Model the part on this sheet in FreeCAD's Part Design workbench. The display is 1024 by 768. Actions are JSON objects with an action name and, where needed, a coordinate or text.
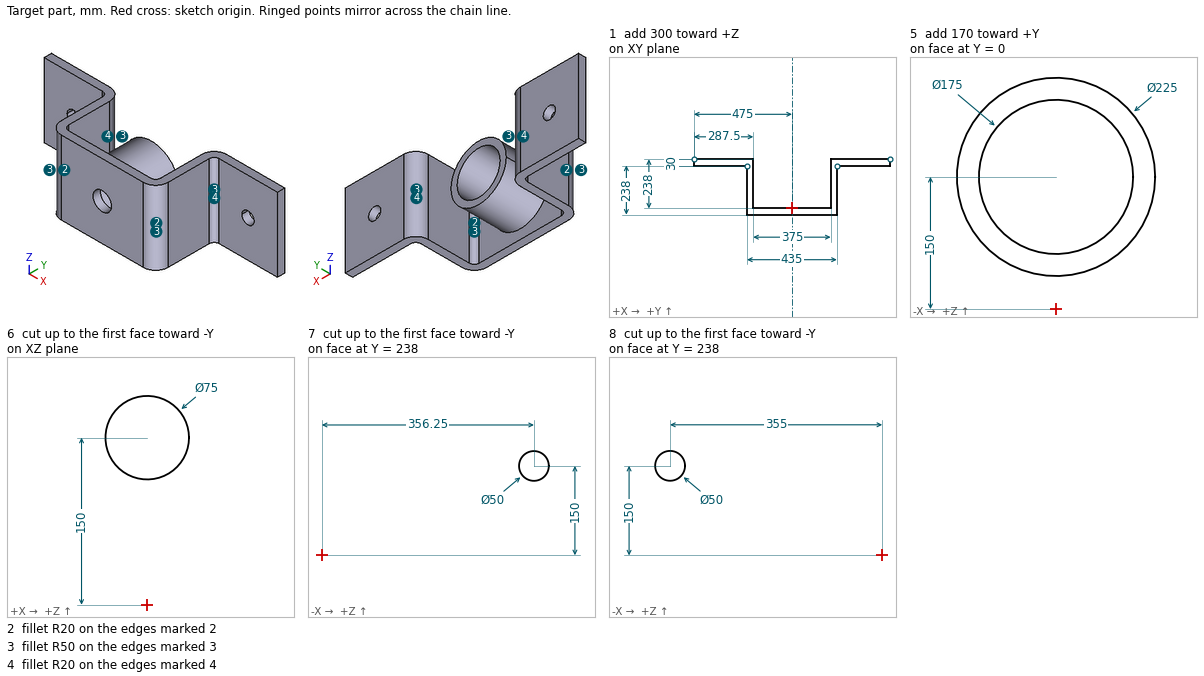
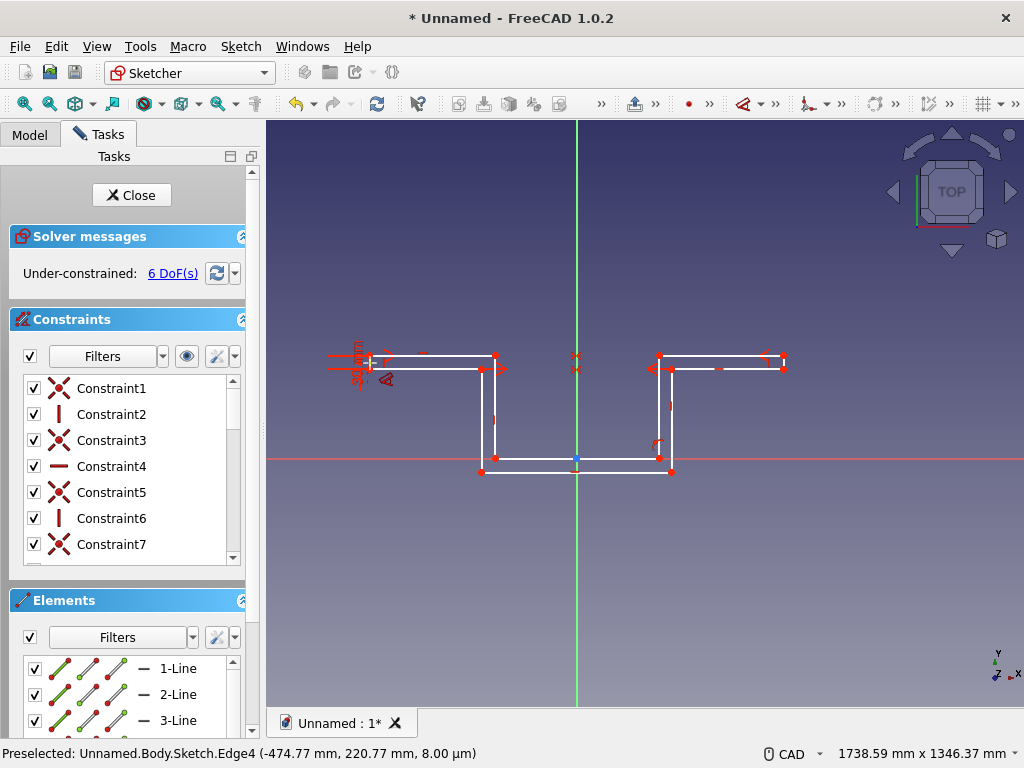
{"action": "left_click", "coordinate": [610, 459]}
{"action": "left_click", "coordinate": [539, 493]}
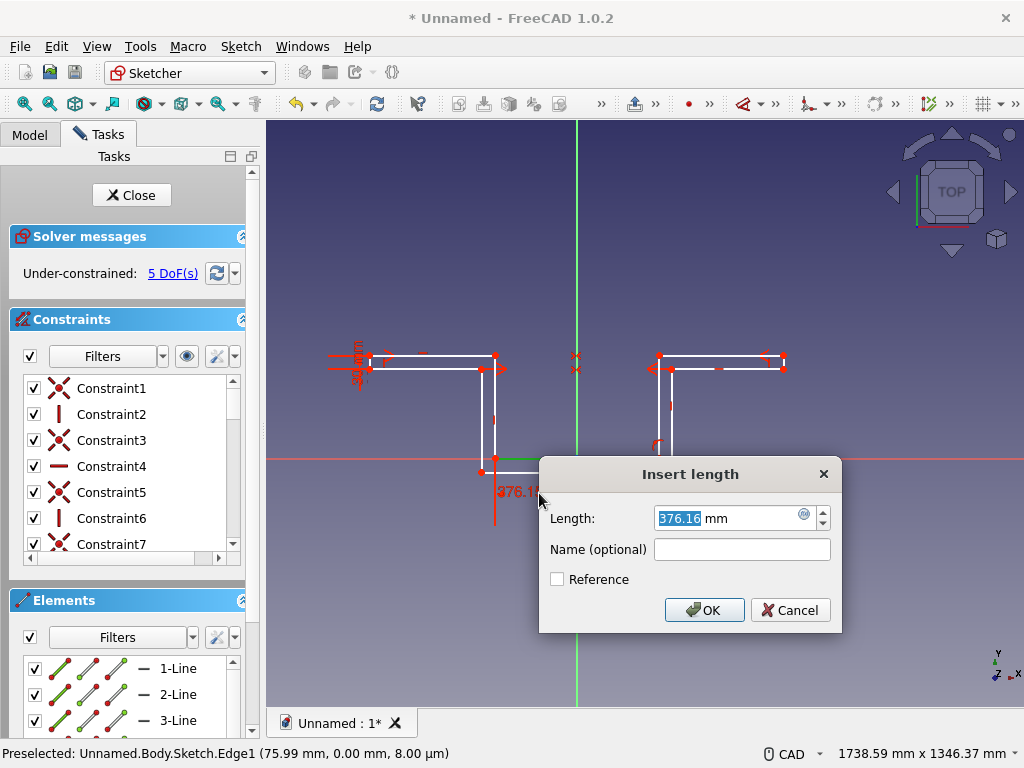
{"action": "type", "text": "375"}
{"action": "key", "text": "Return"}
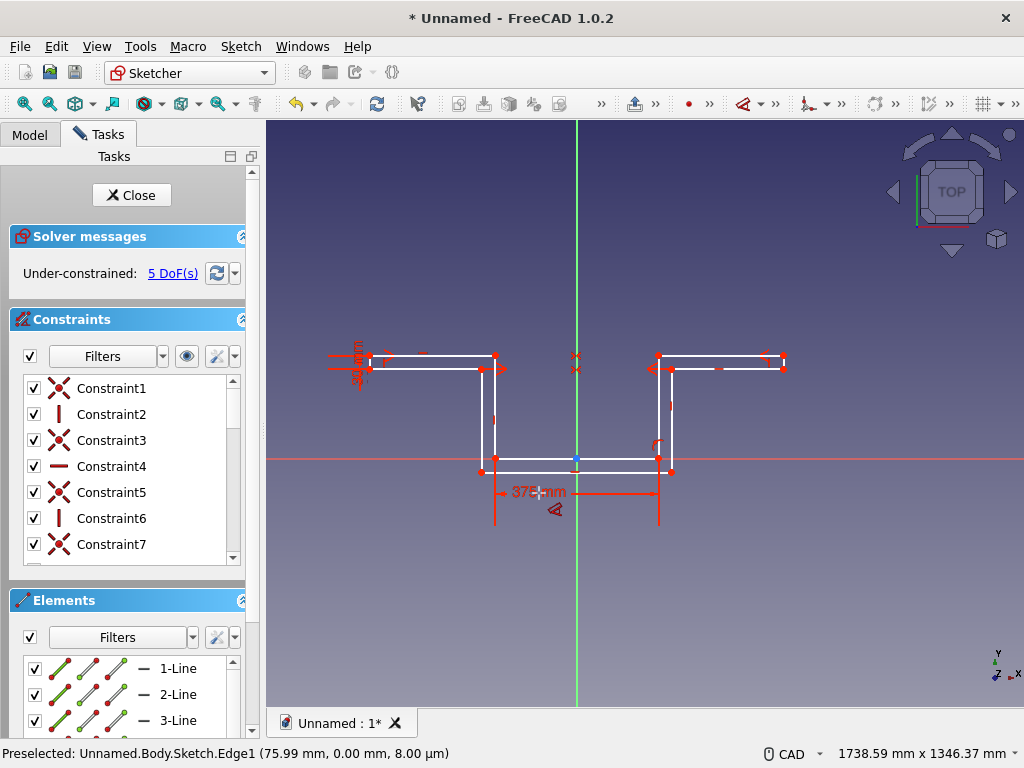
{"action": "left_click", "coordinate": [495, 428]}
{"action": "left_click", "coordinate": [461, 407]}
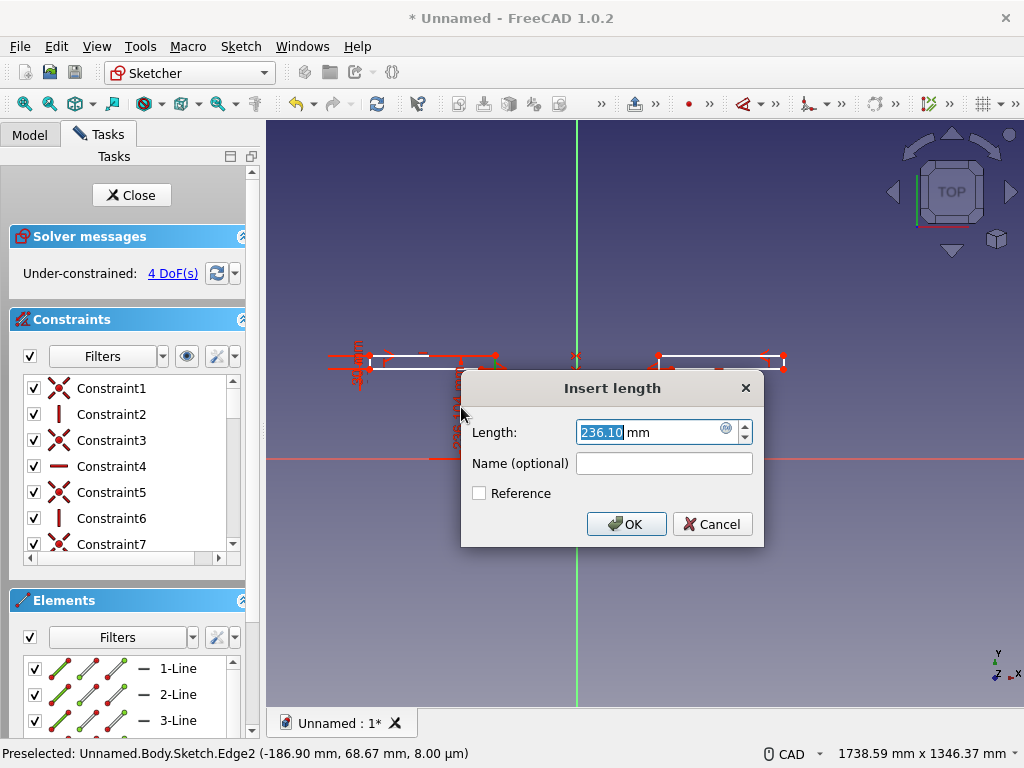
{"action": "type", "text": "238"}
{"action": "key", "text": "Return"}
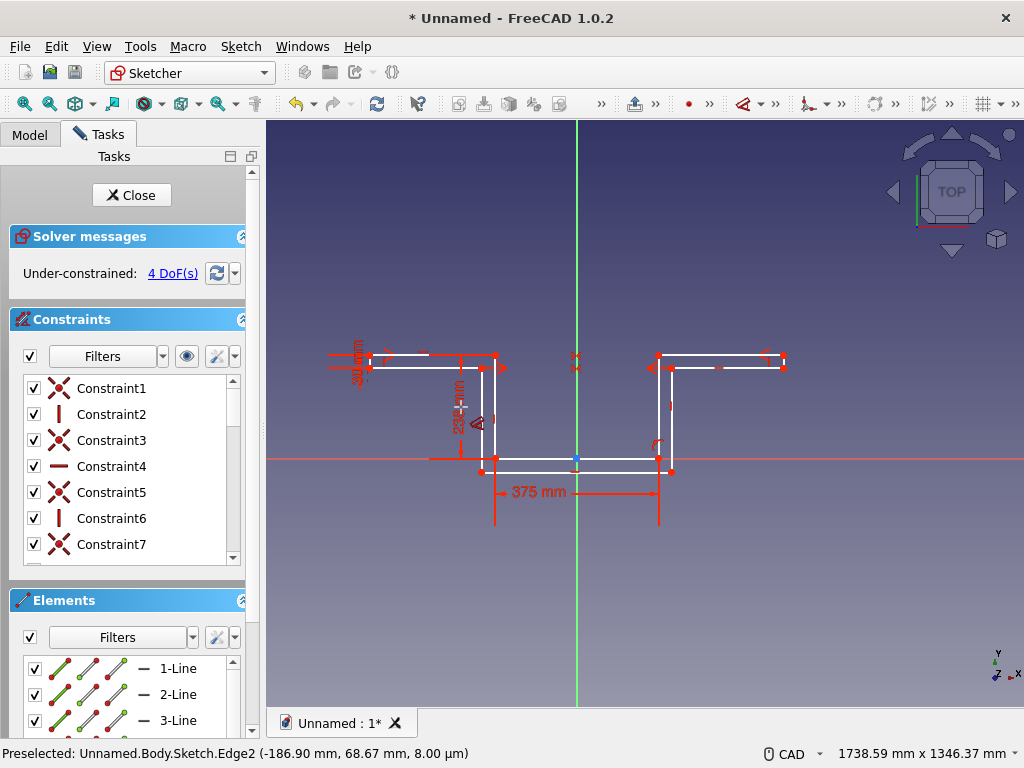
{"action": "left_click", "coordinate": [482, 400]}
{"action": "left_click", "coordinate": [448, 445]}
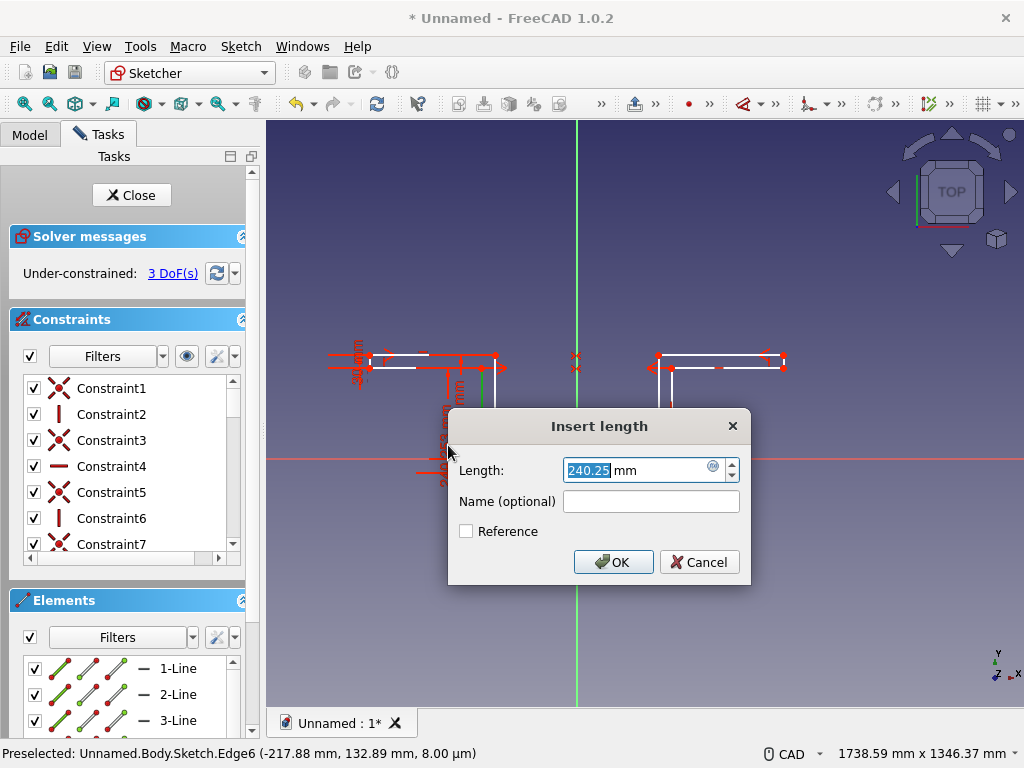
{"action": "type", "text": "238"}
{"action": "key", "text": "Return"}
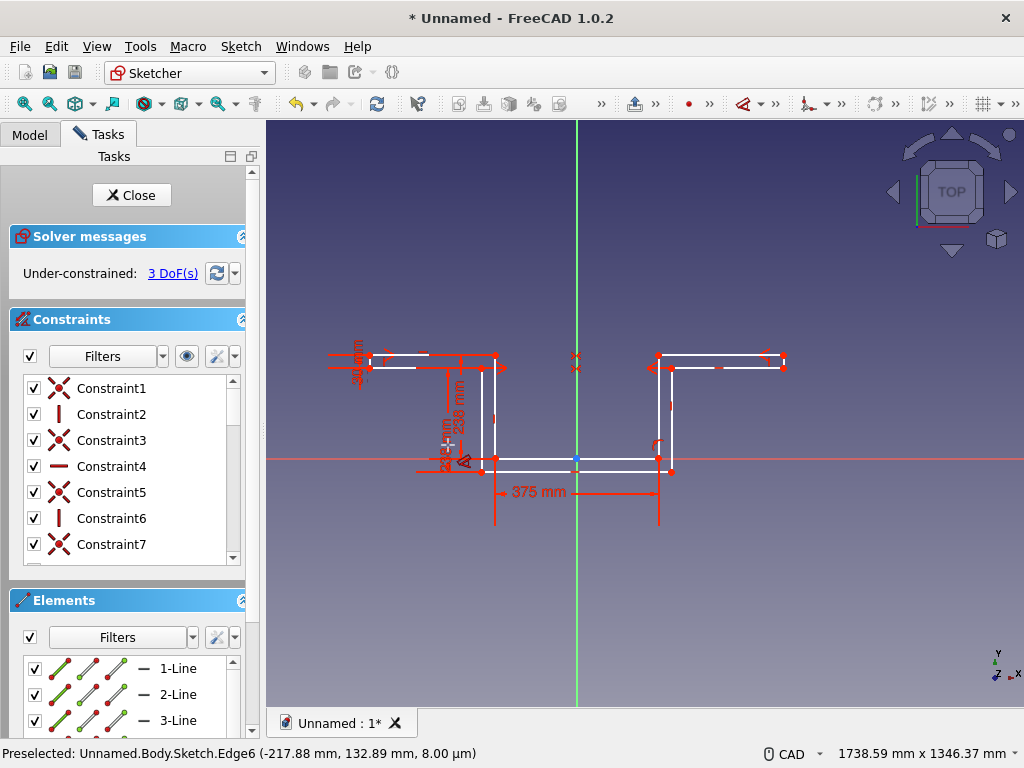
{"action": "left_click", "coordinate": [539, 472]}
{"action": "left_click", "coordinate": [621, 506]}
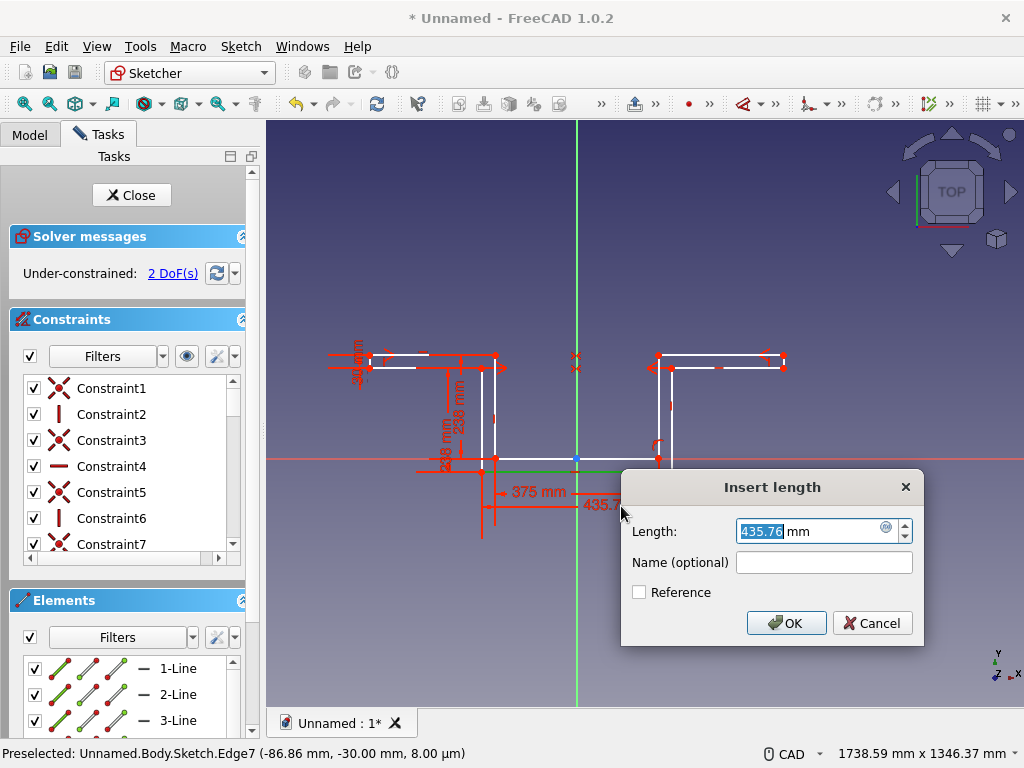
{"action": "type", "text": "435"}
{"action": "key", "text": "Return"}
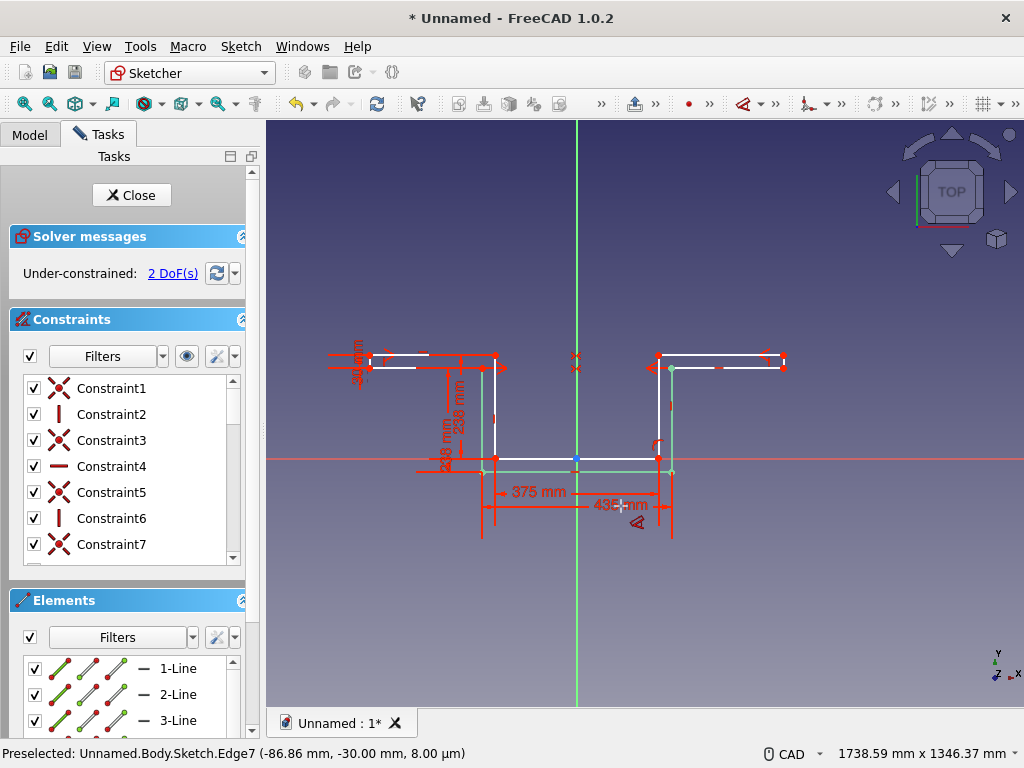
{"action": "left_click", "coordinate": [370, 355]}
{"action": "left_click", "coordinate": [473, 321]}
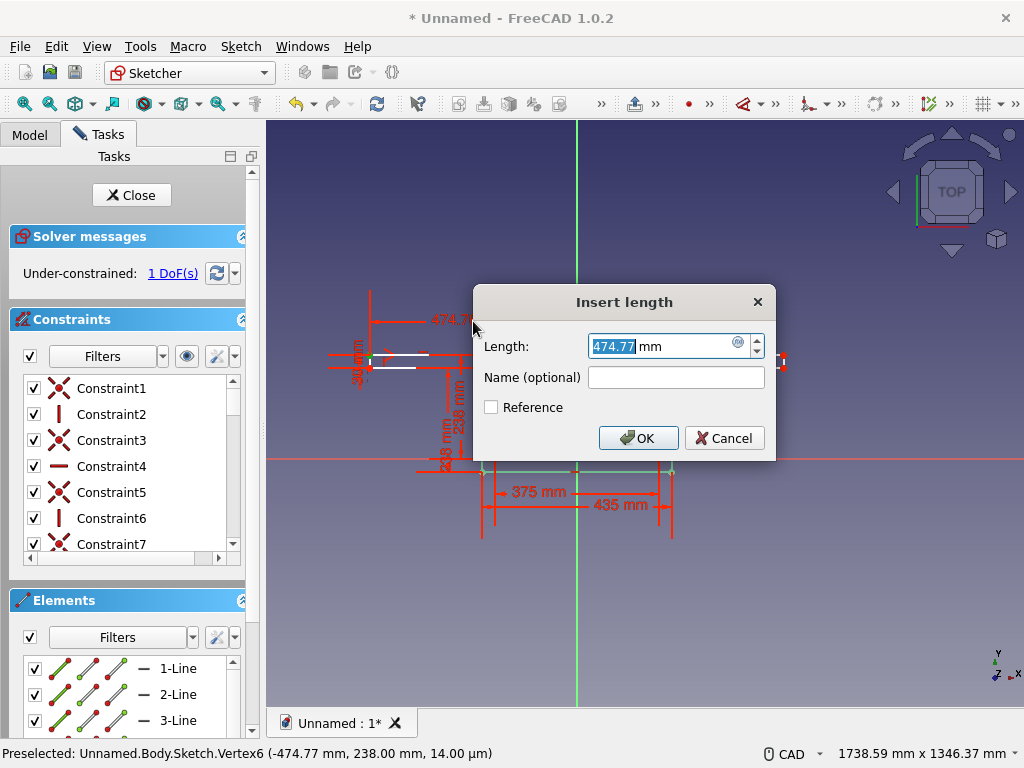
{"action": "type", "text": "475"}
{"action": "key", "text": "Return"}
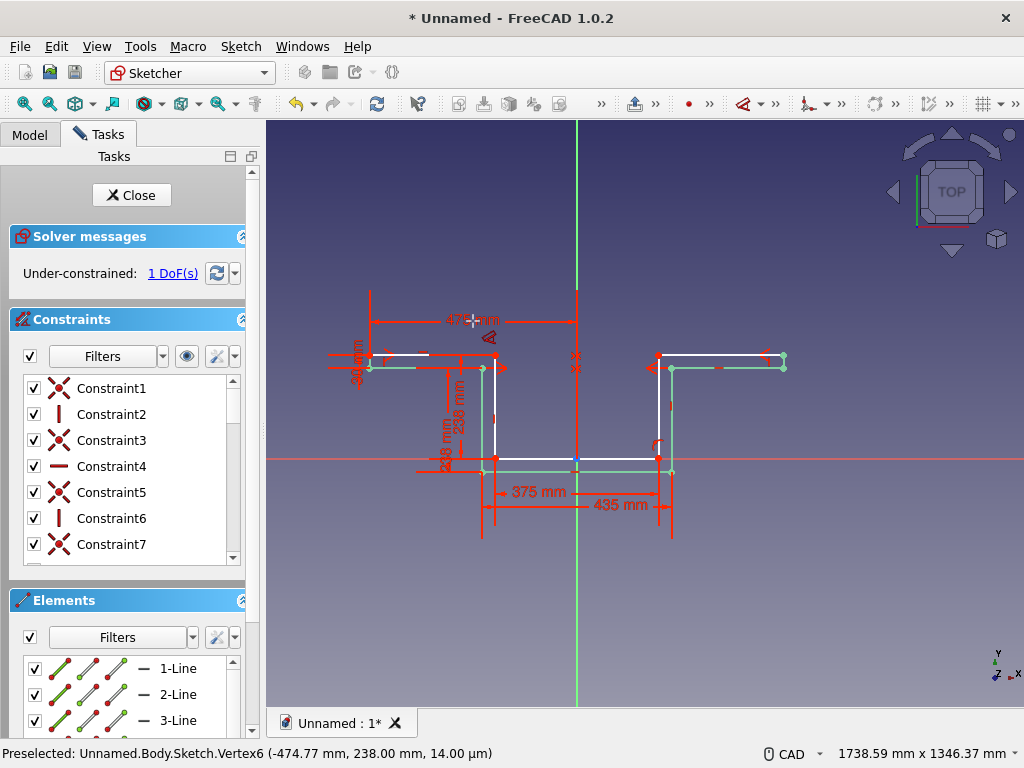
{"action": "left_click", "coordinate": [458, 355]}
{"action": "left_click", "coordinate": [389, 321]}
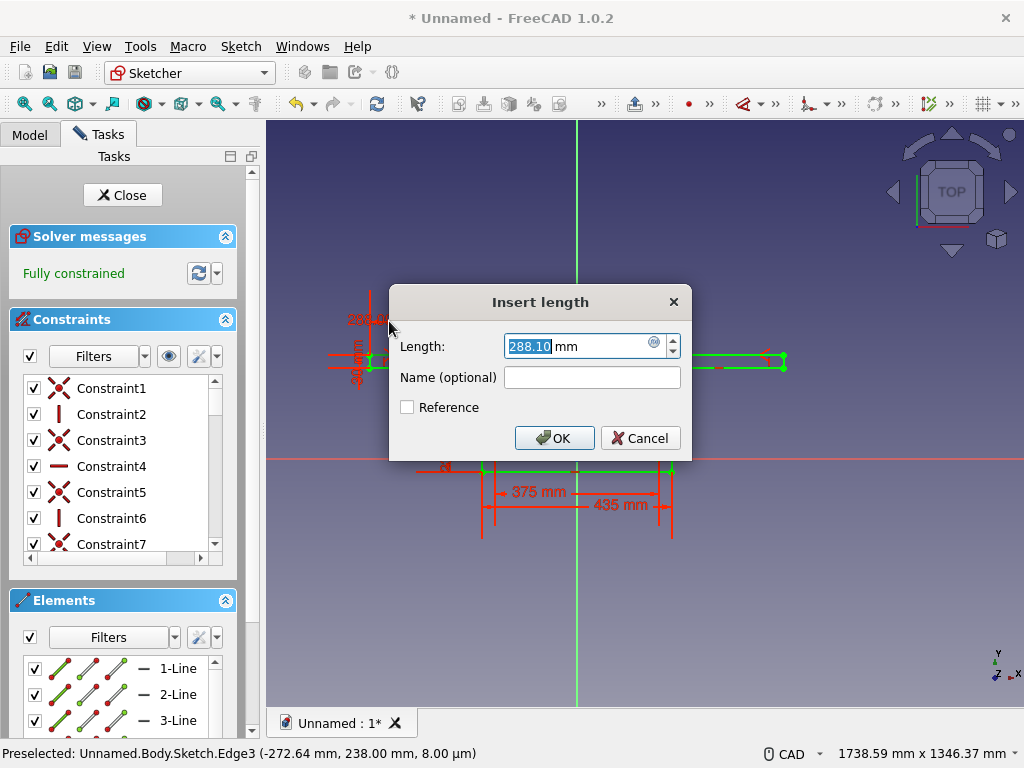
{"action": "type", "text": "287.5"}
{"action": "key", "text": "Return"}
{"action": "key", "text": "Escape"}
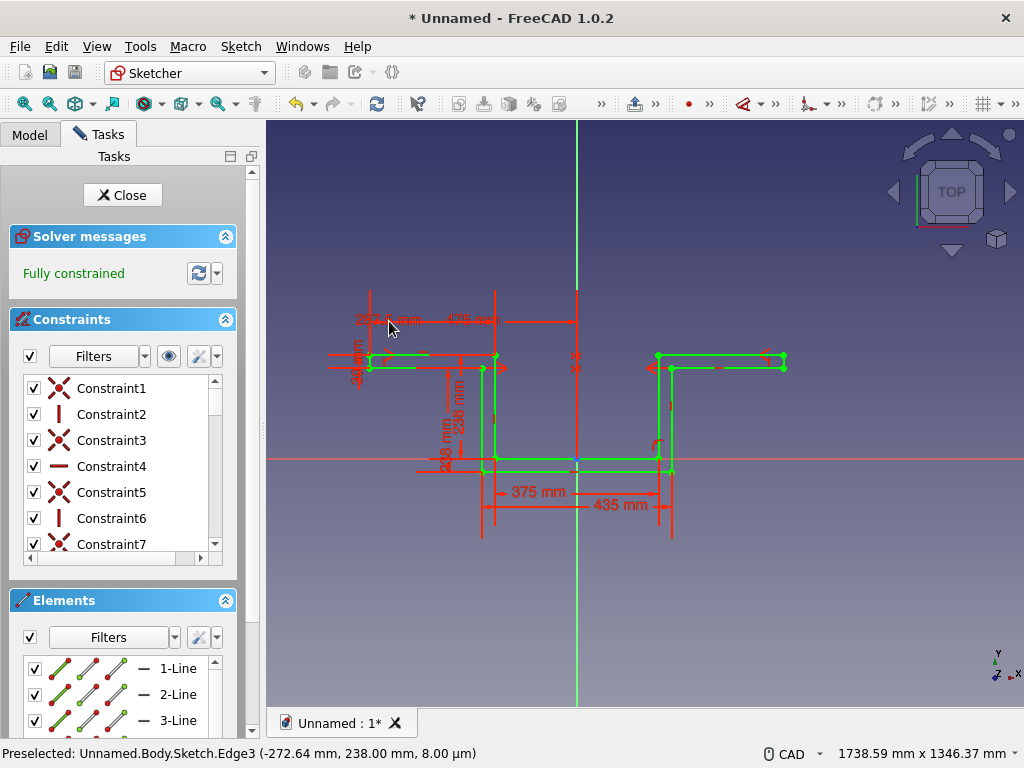
{"action": "left_click", "coordinate": [123, 195]}